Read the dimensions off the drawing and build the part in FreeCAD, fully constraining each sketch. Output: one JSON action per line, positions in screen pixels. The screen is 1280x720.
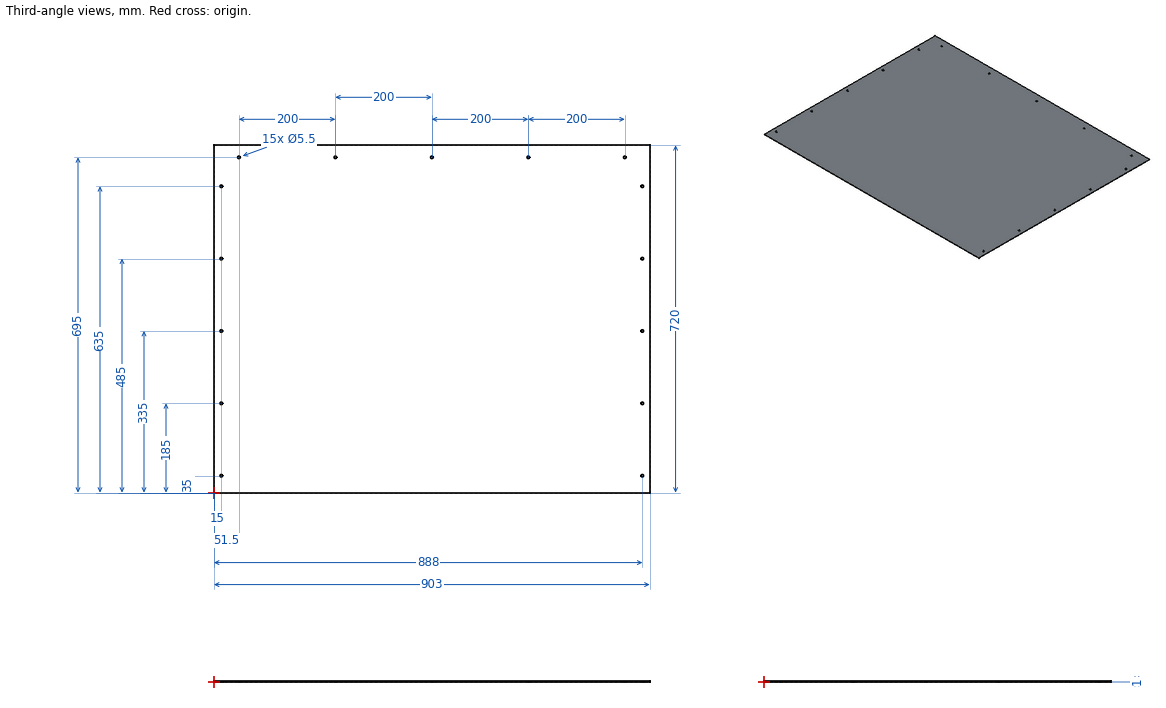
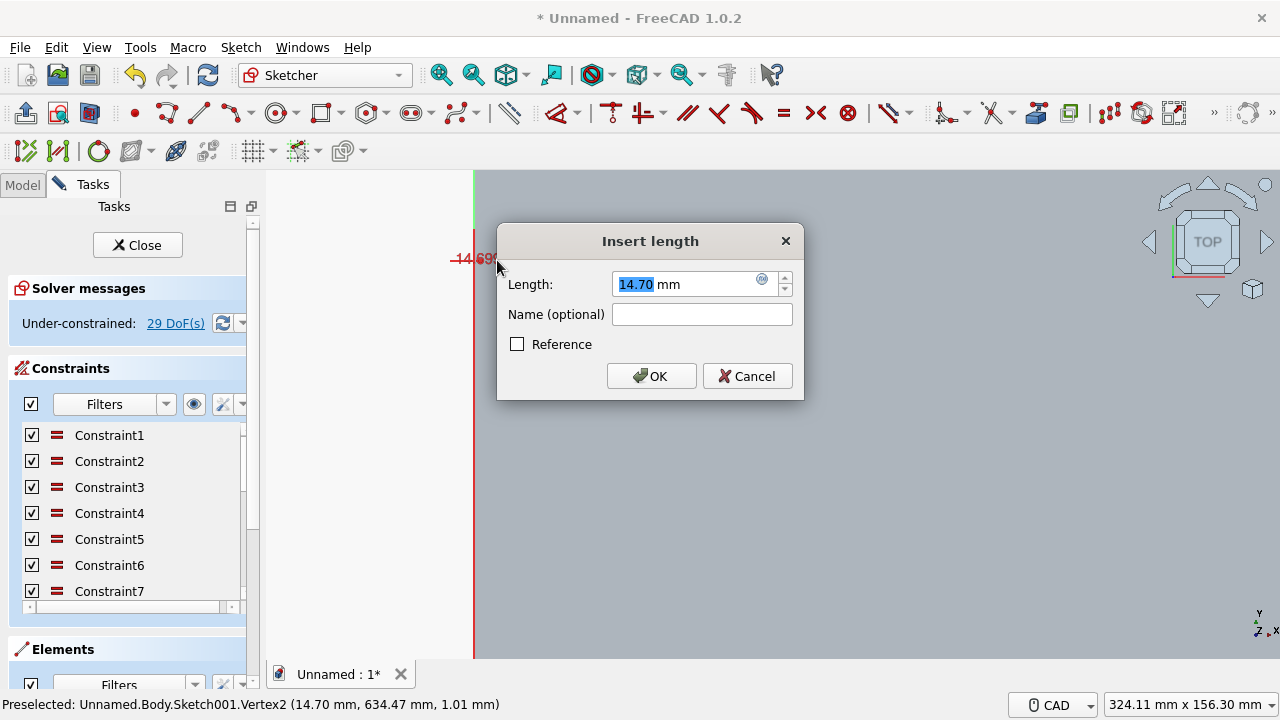
{"action": "type", "text": "15"}
{"action": "key", "text": "Return"}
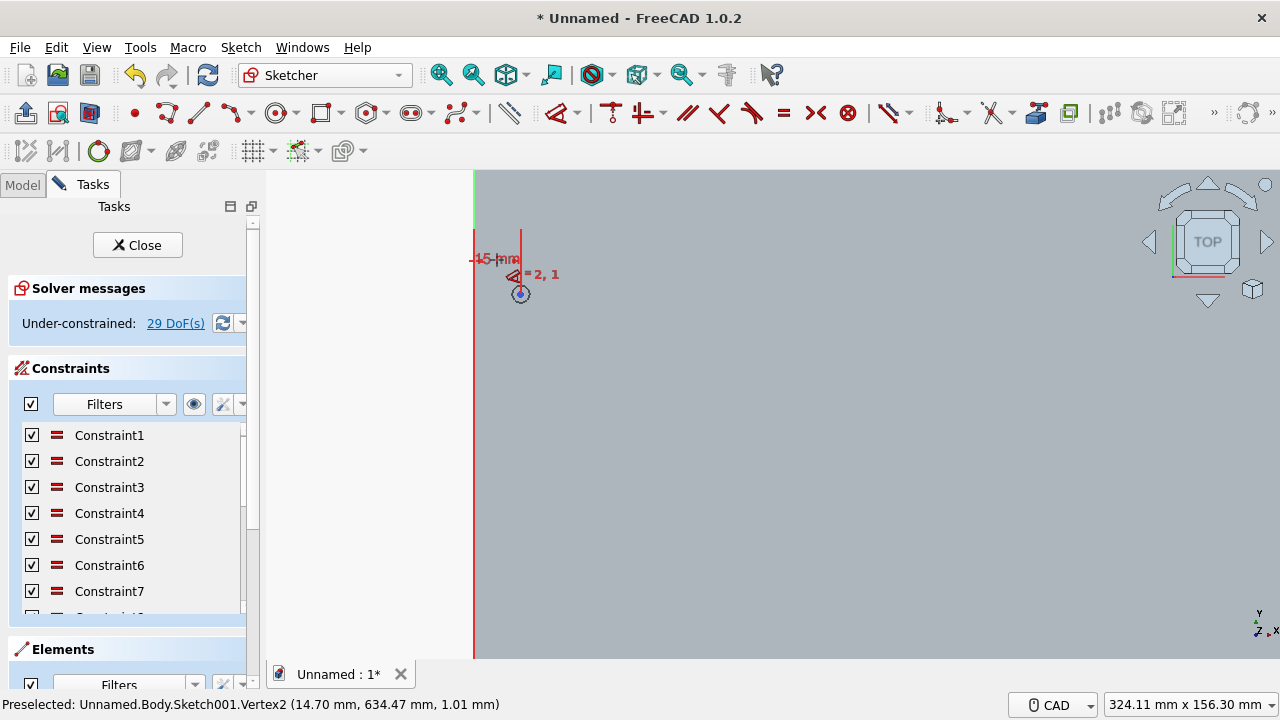
{"action": "scroll", "coordinate": [522, 293], "scroll_direction": "down", "scroll_amount": 10}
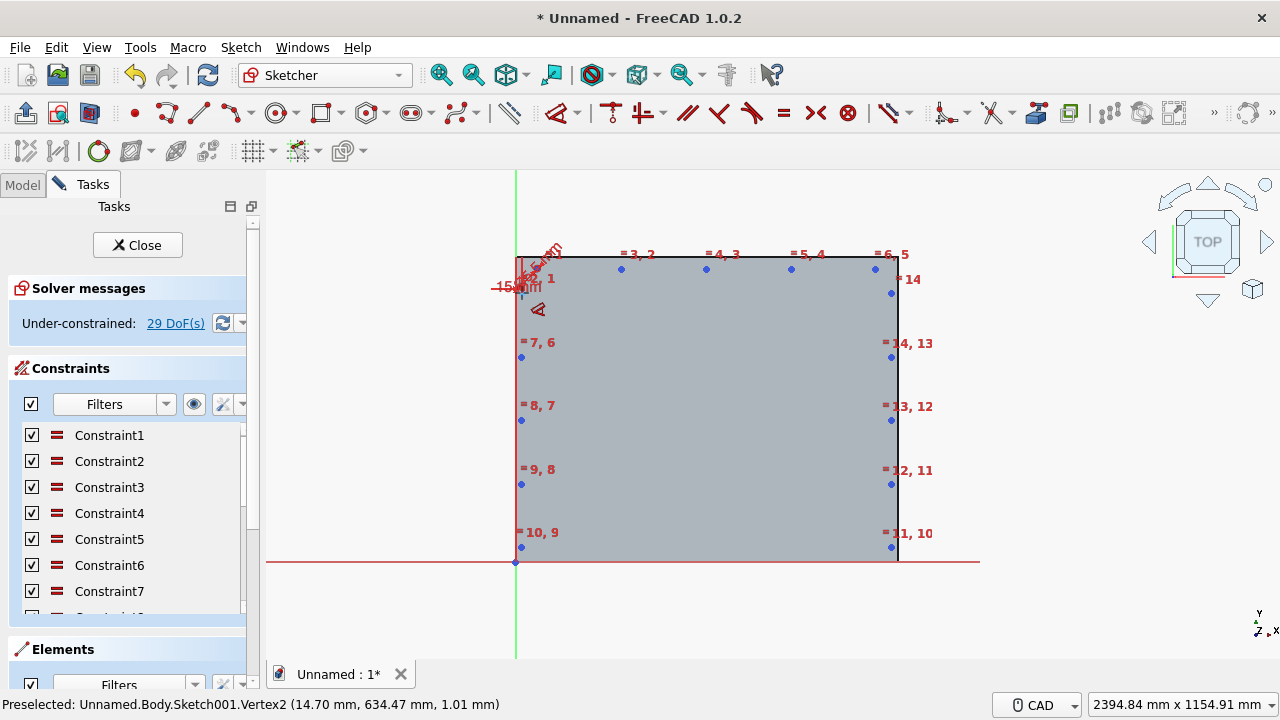
{"action": "scroll", "coordinate": [522, 357], "scroll_direction": "up", "scroll_amount": 10}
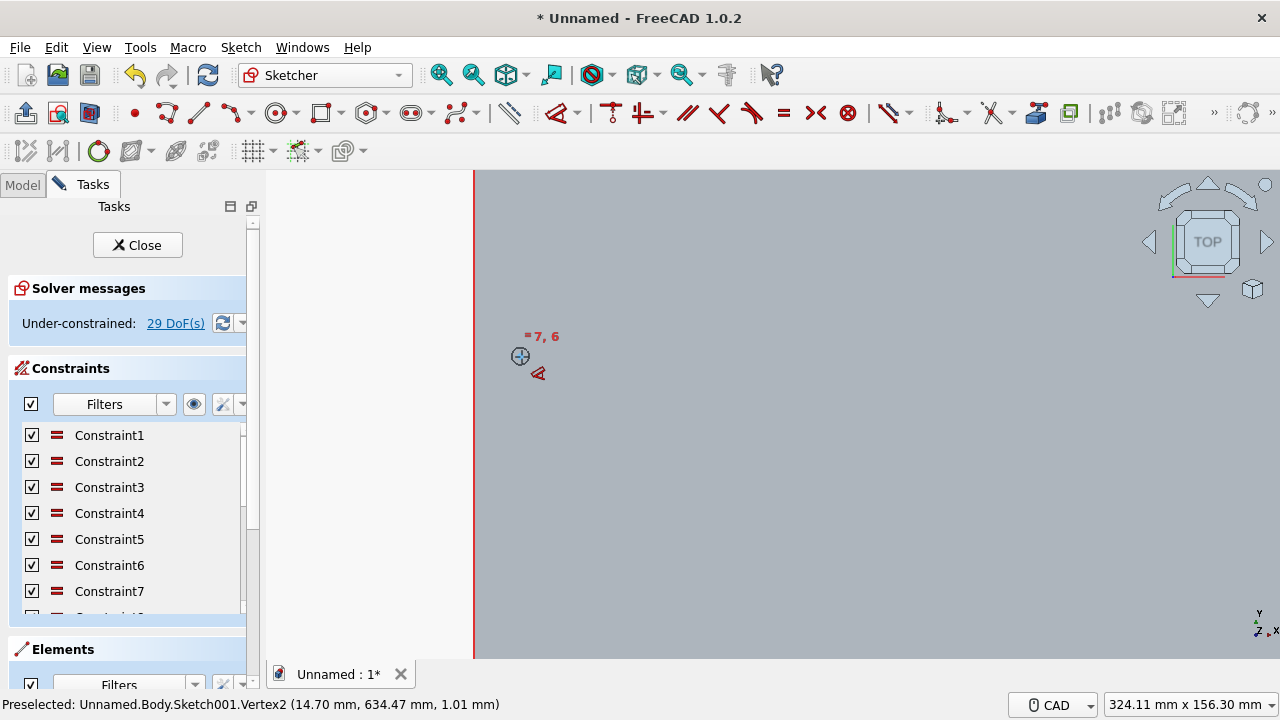
{"action": "left_click", "coordinate": [520, 356]}
{"action": "left_click", "coordinate": [497, 322]}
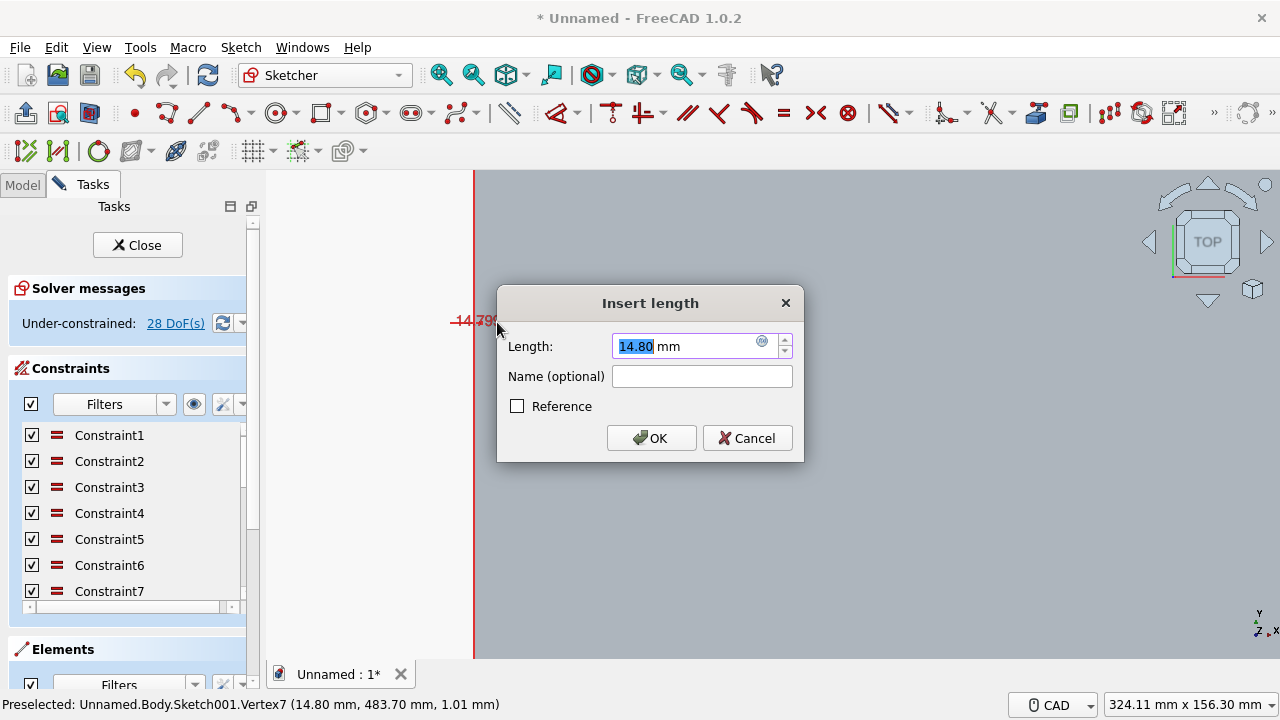
{"action": "type", "text": "15"}
{"action": "key", "text": "Return"}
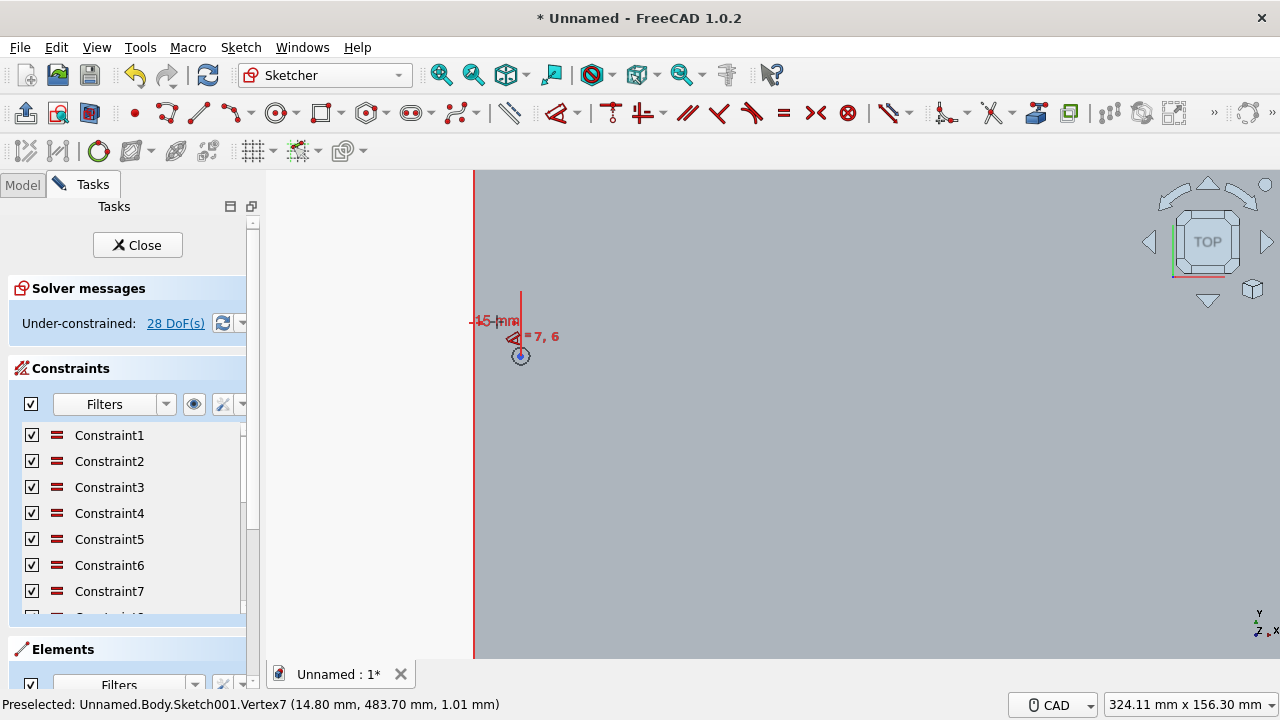
{"action": "scroll", "coordinate": [522, 358], "scroll_direction": "down", "scroll_amount": 10}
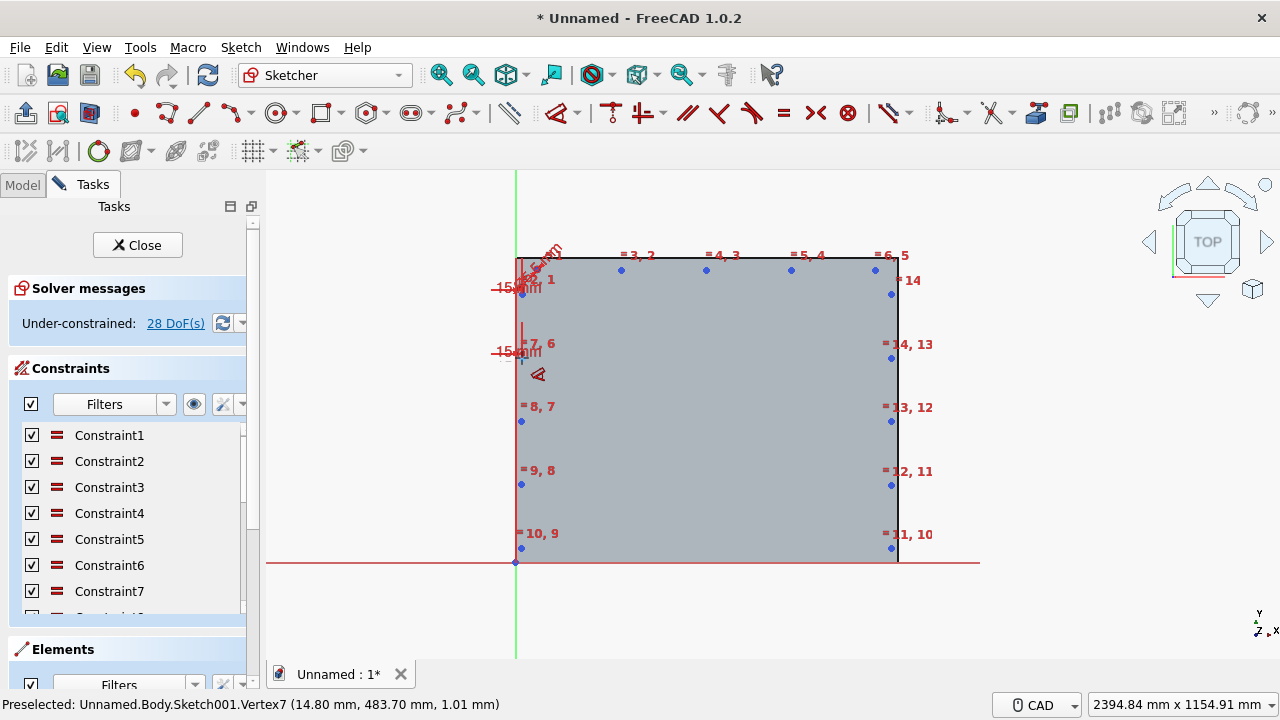
{"action": "scroll", "coordinate": [522, 421], "scroll_direction": "up", "scroll_amount": 10}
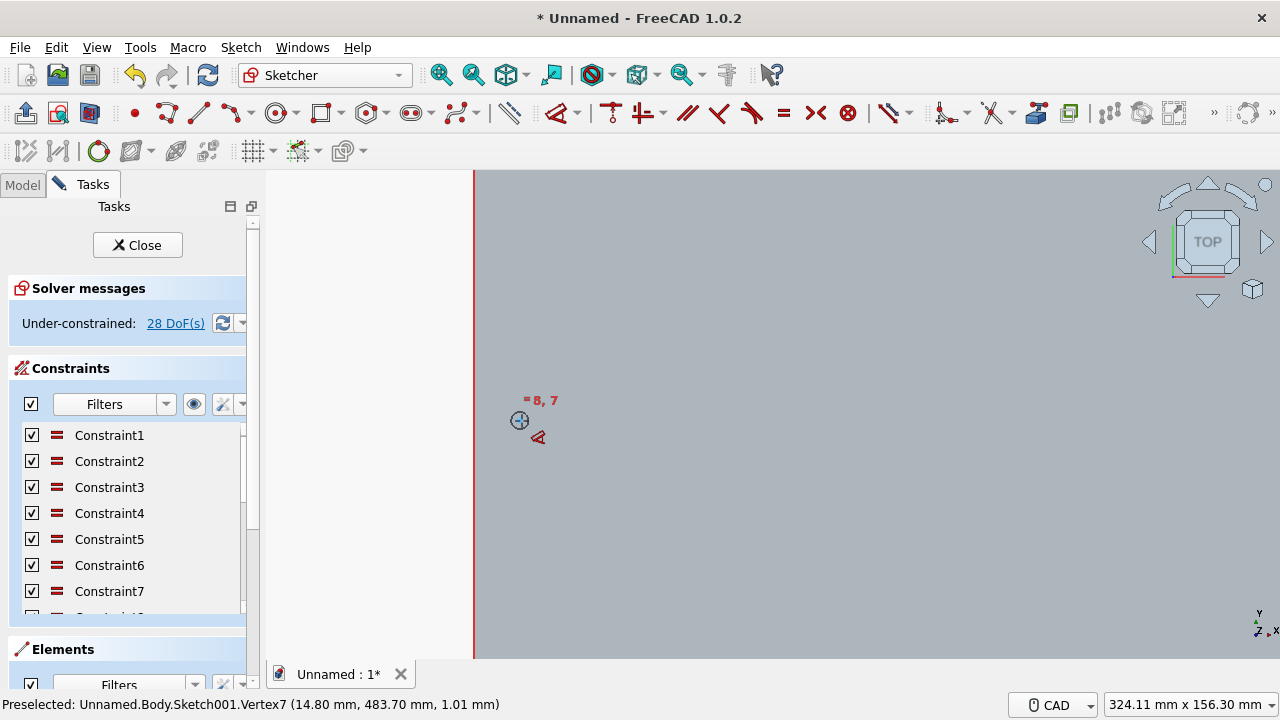
{"action": "left_click", "coordinate": [520, 421]}
{"action": "left_click", "coordinate": [497, 387]}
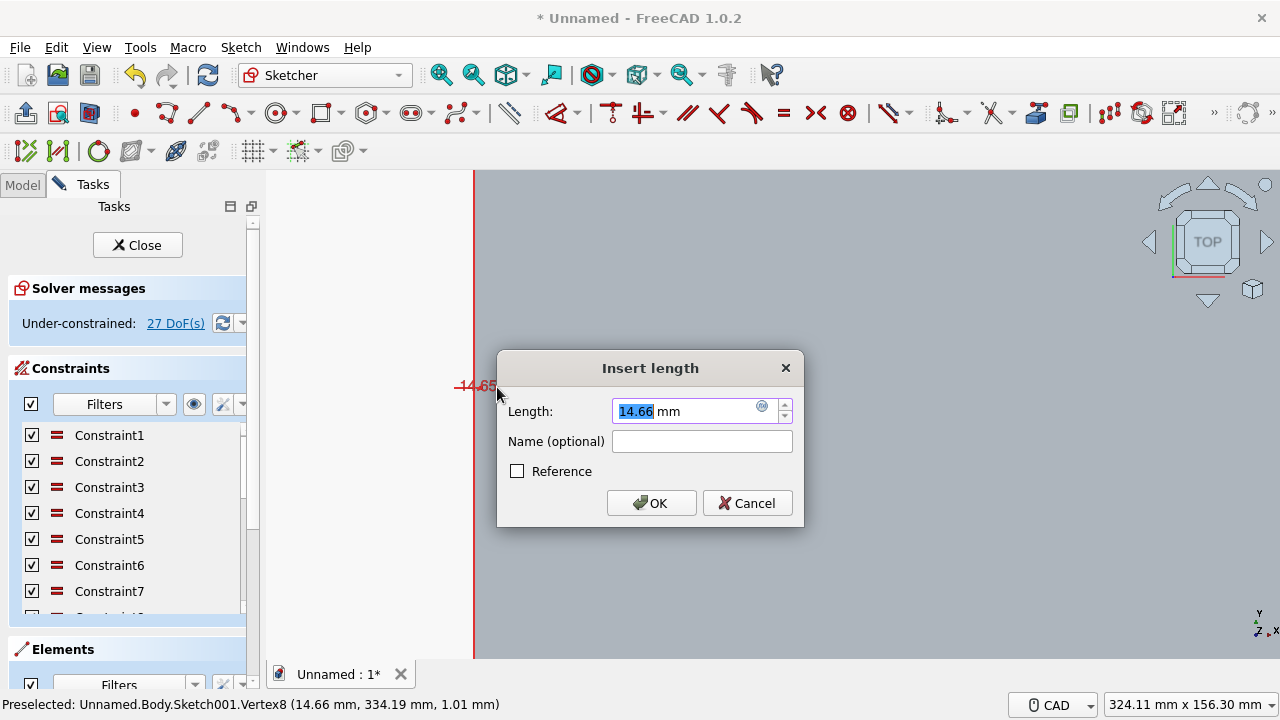
{"action": "type", "text": "15"}
{"action": "key", "text": "Return"}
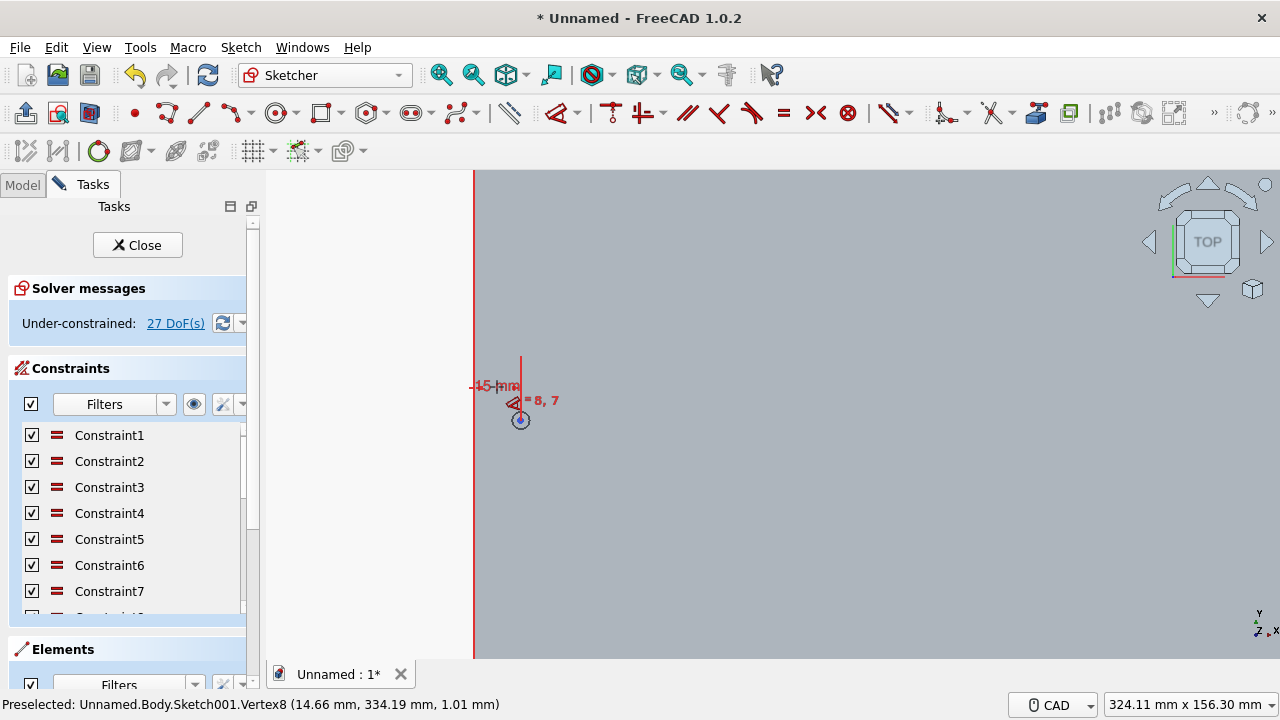
{"action": "scroll", "coordinate": [522, 421], "scroll_direction": "down", "scroll_amount": 10}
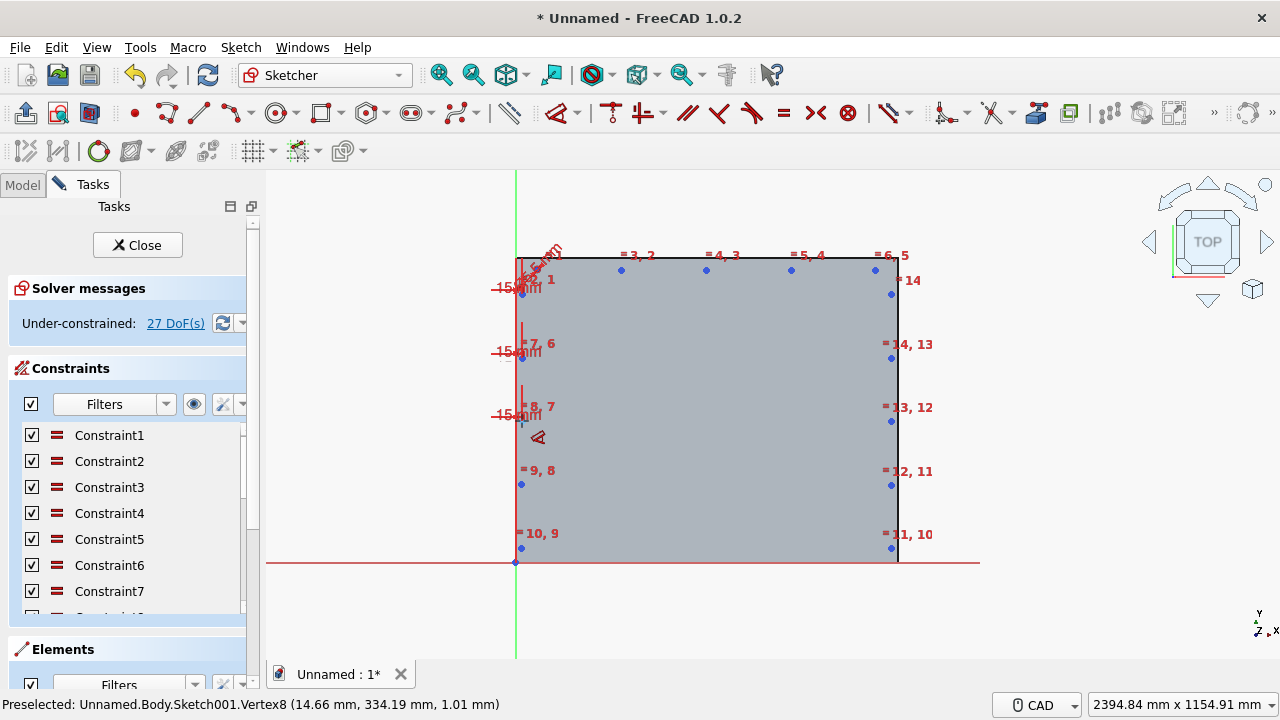
{"action": "scroll", "coordinate": [522, 485], "scroll_direction": "up", "scroll_amount": 10}